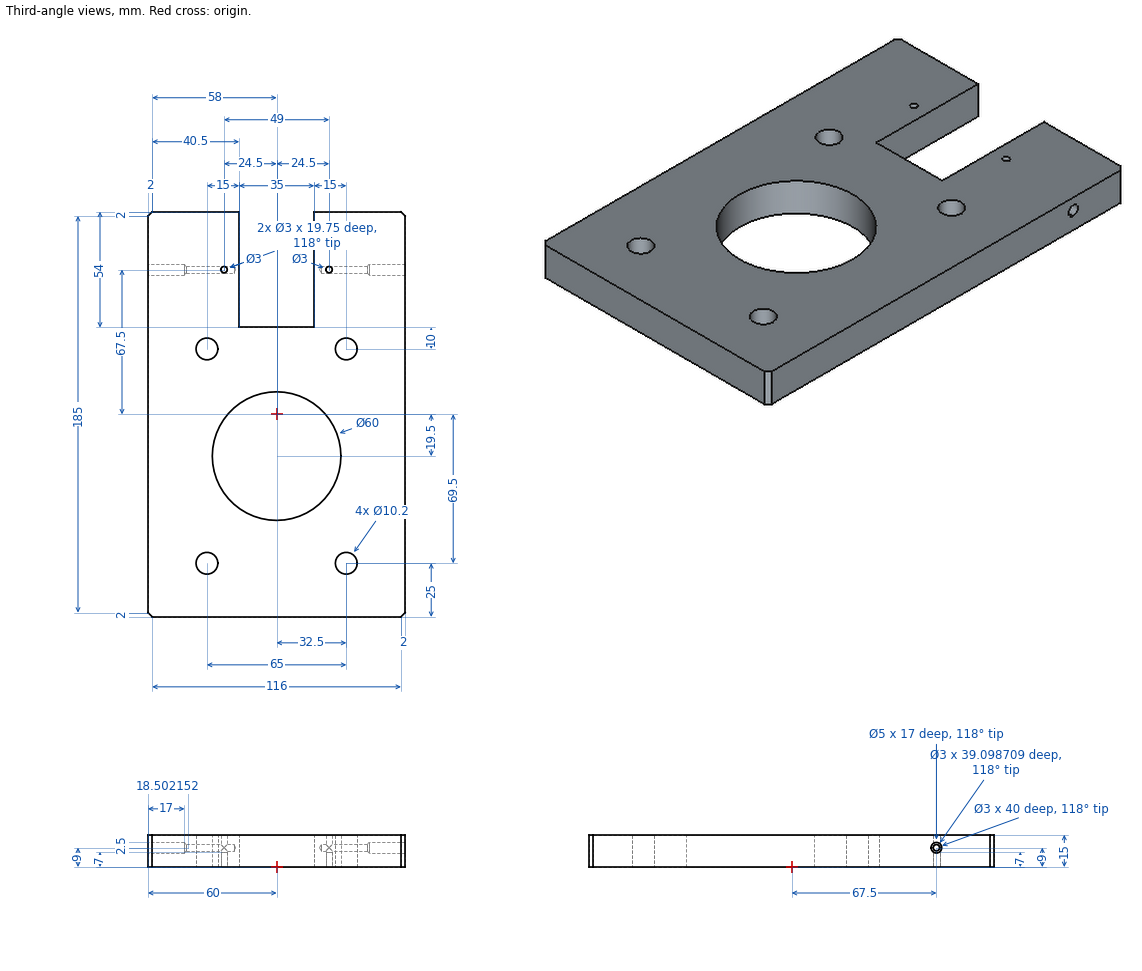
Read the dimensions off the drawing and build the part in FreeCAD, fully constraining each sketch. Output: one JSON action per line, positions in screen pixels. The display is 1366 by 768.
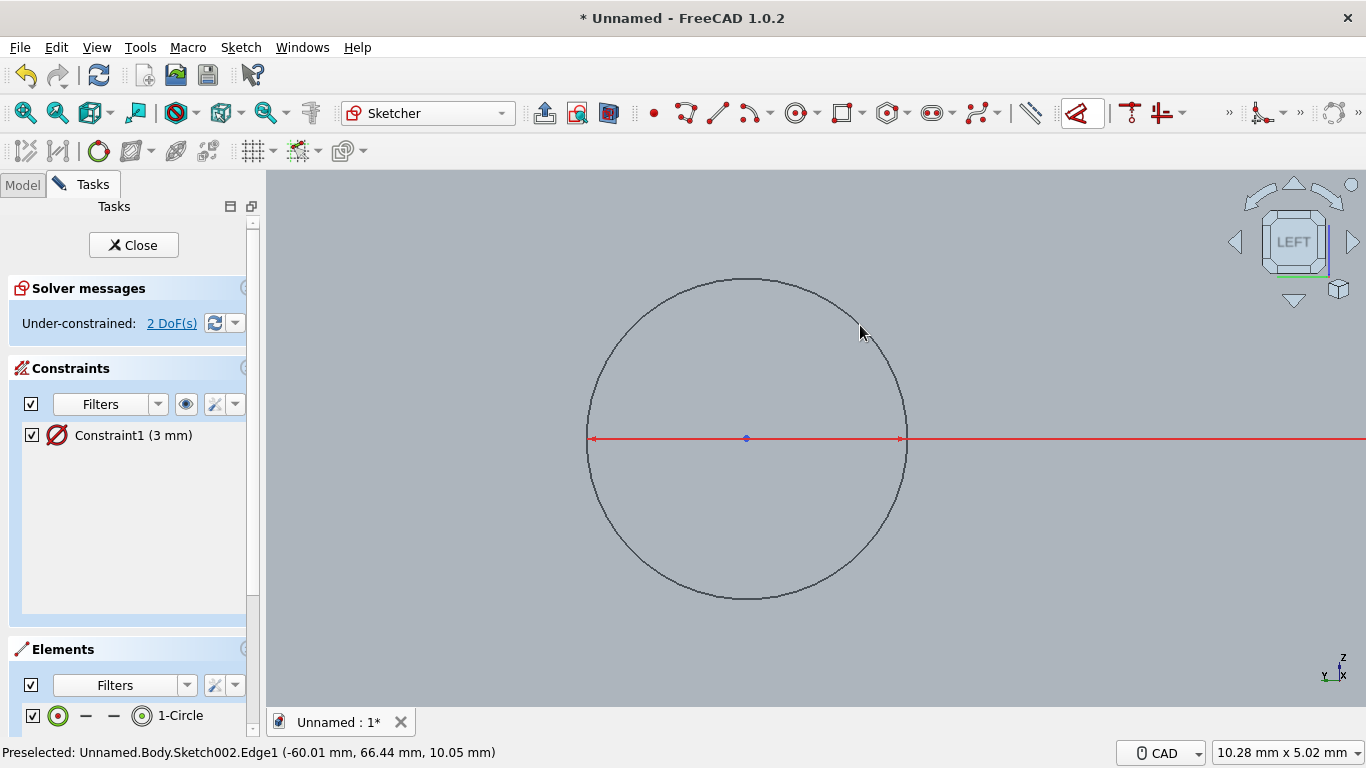
{"action": "left_click", "coordinate": [747, 439]}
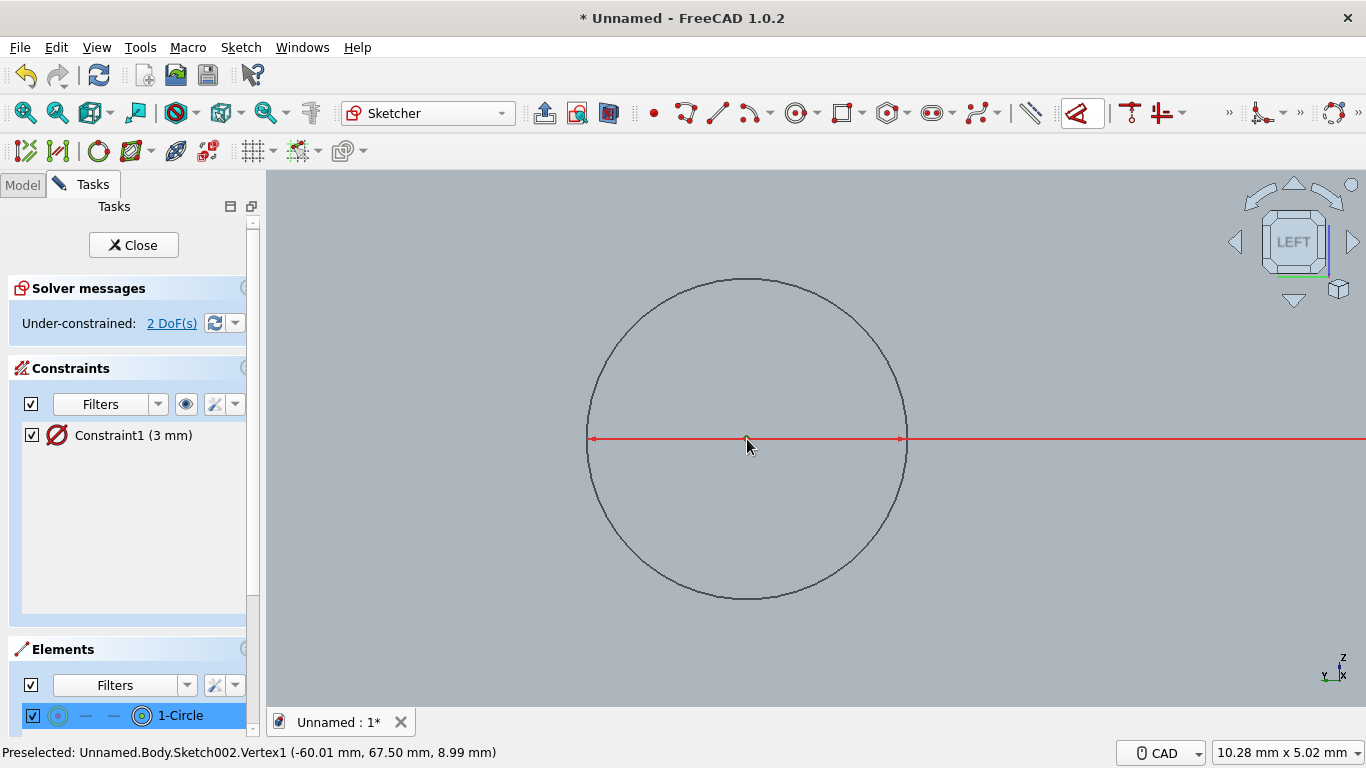
{"action": "left_click", "coordinate": [1098, 114]}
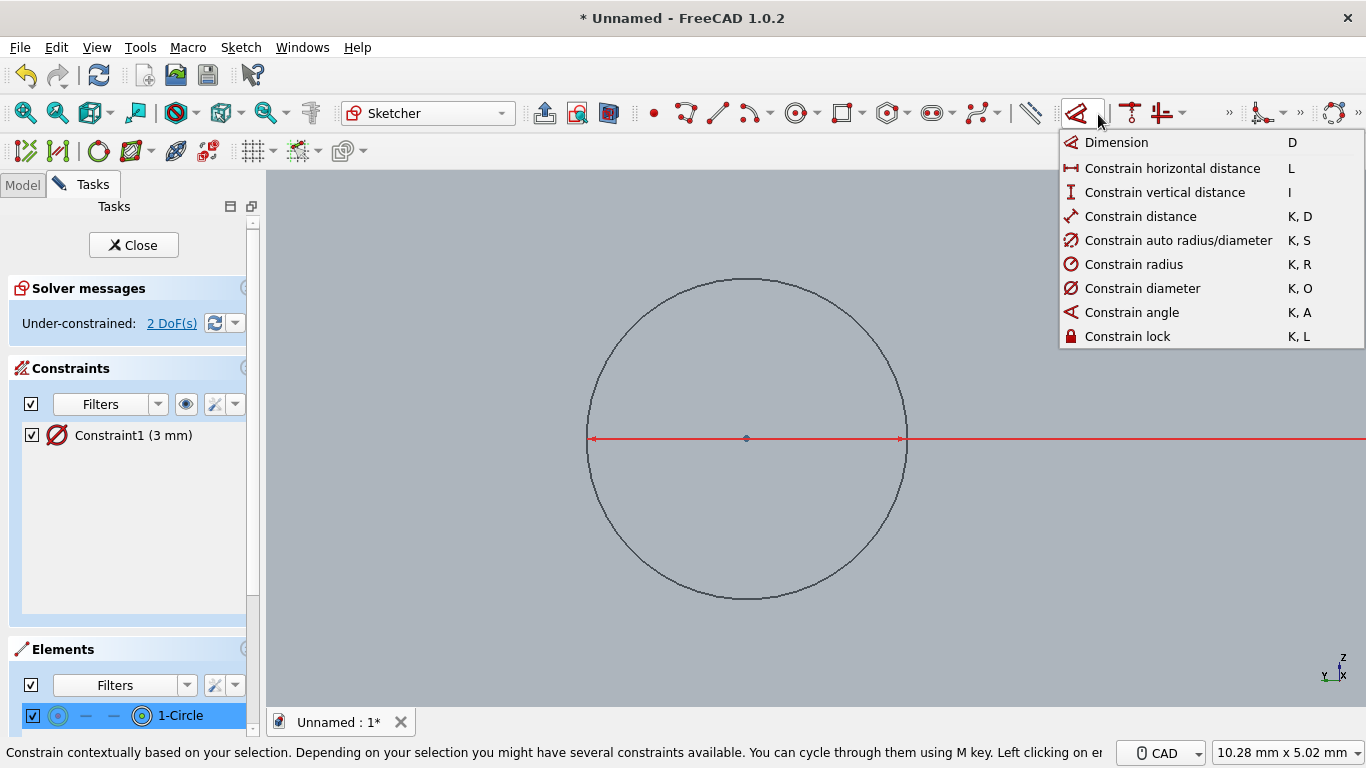
{"action": "left_click", "coordinate": [1212, 192]}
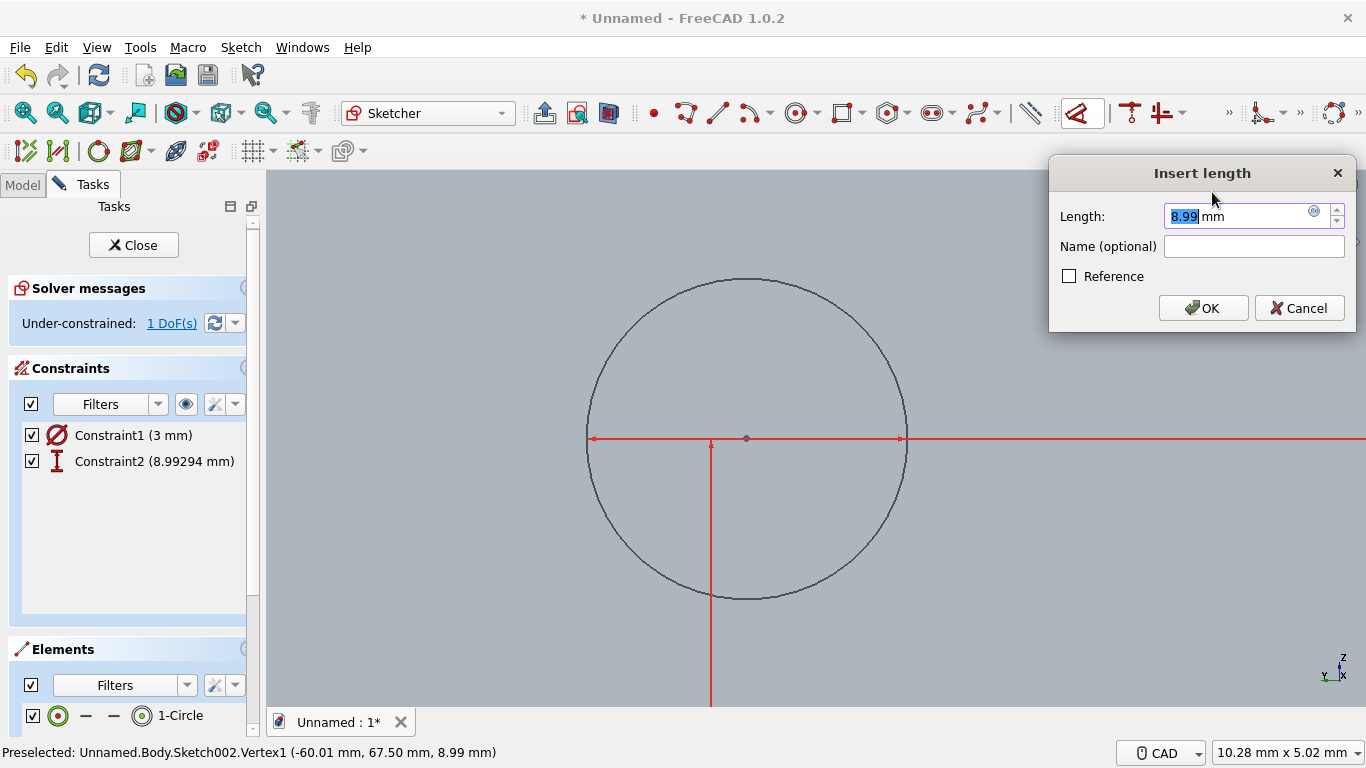
{"action": "type", "text": "9"}
{"action": "key", "text": "Return"}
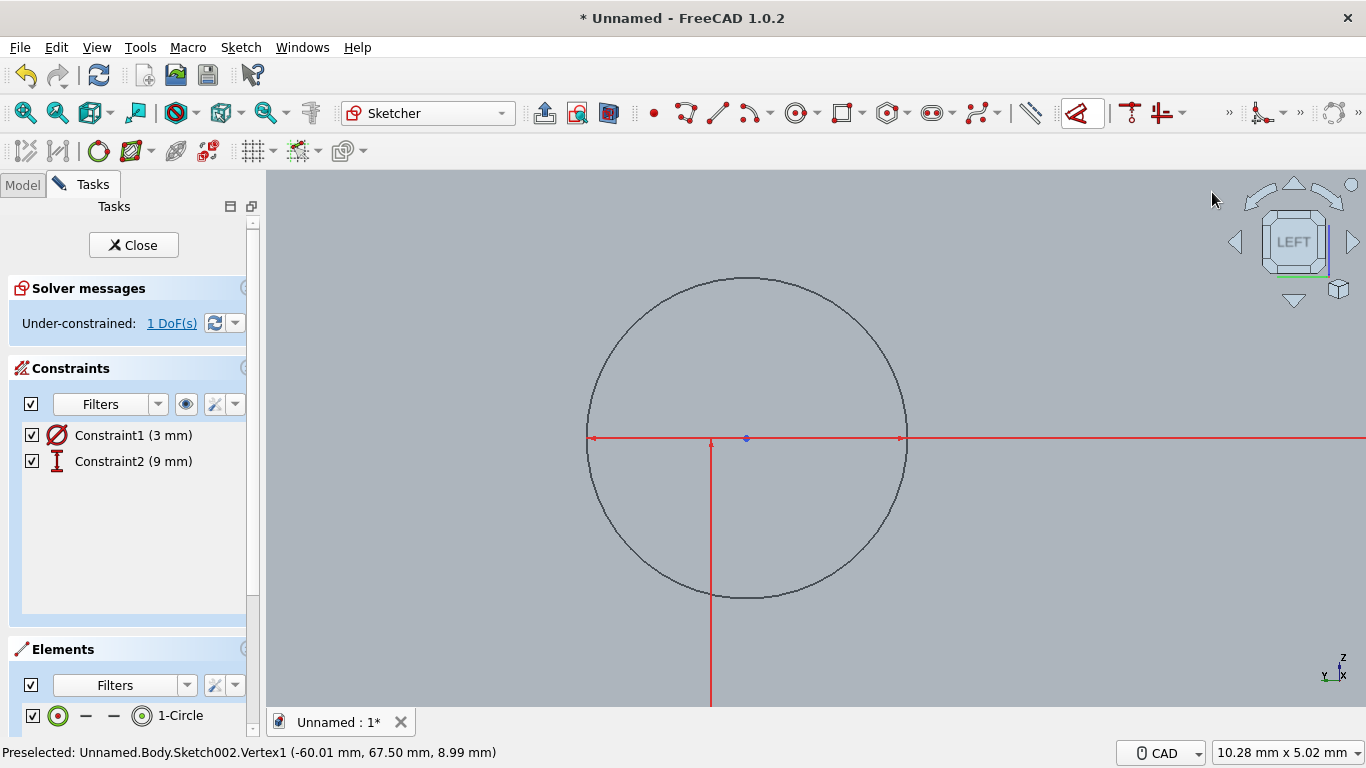
{"action": "left_click", "coordinate": [747, 438]}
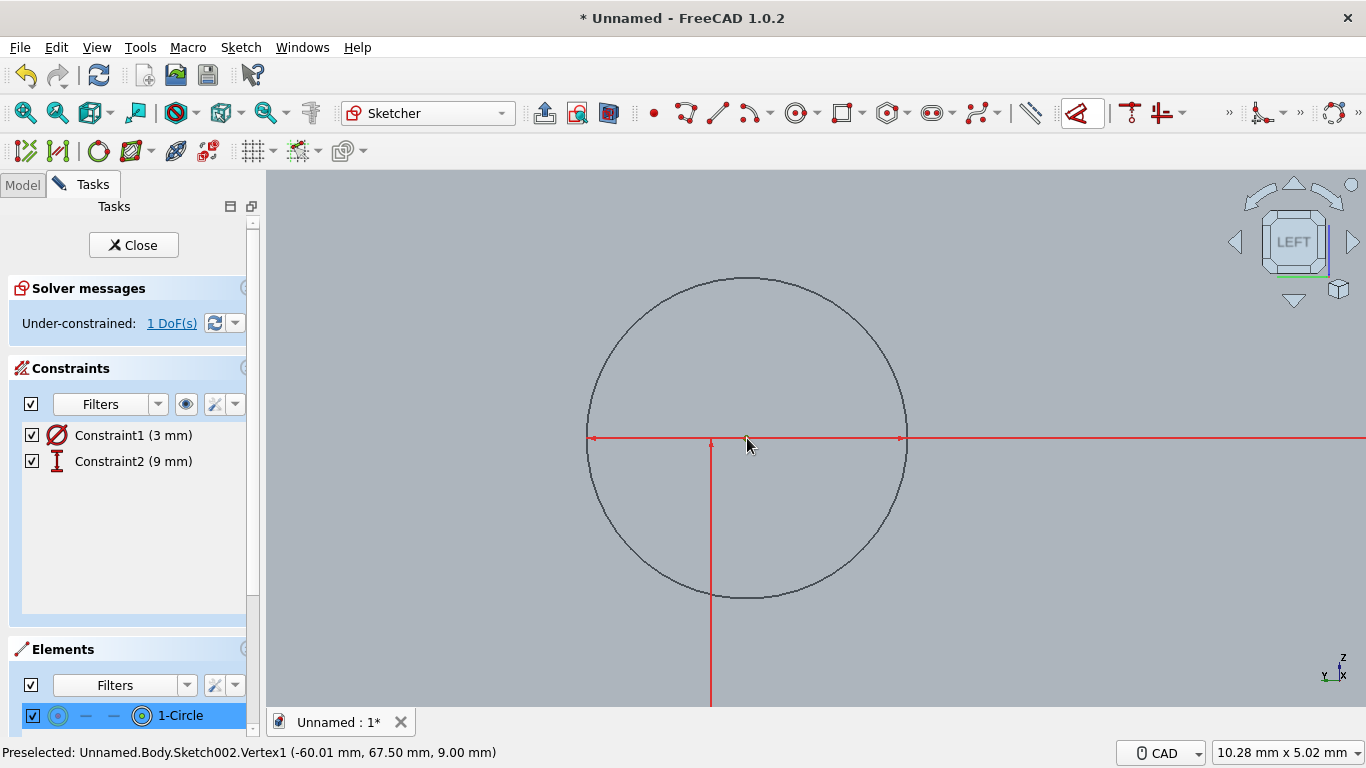
{"action": "key", "text": "l"}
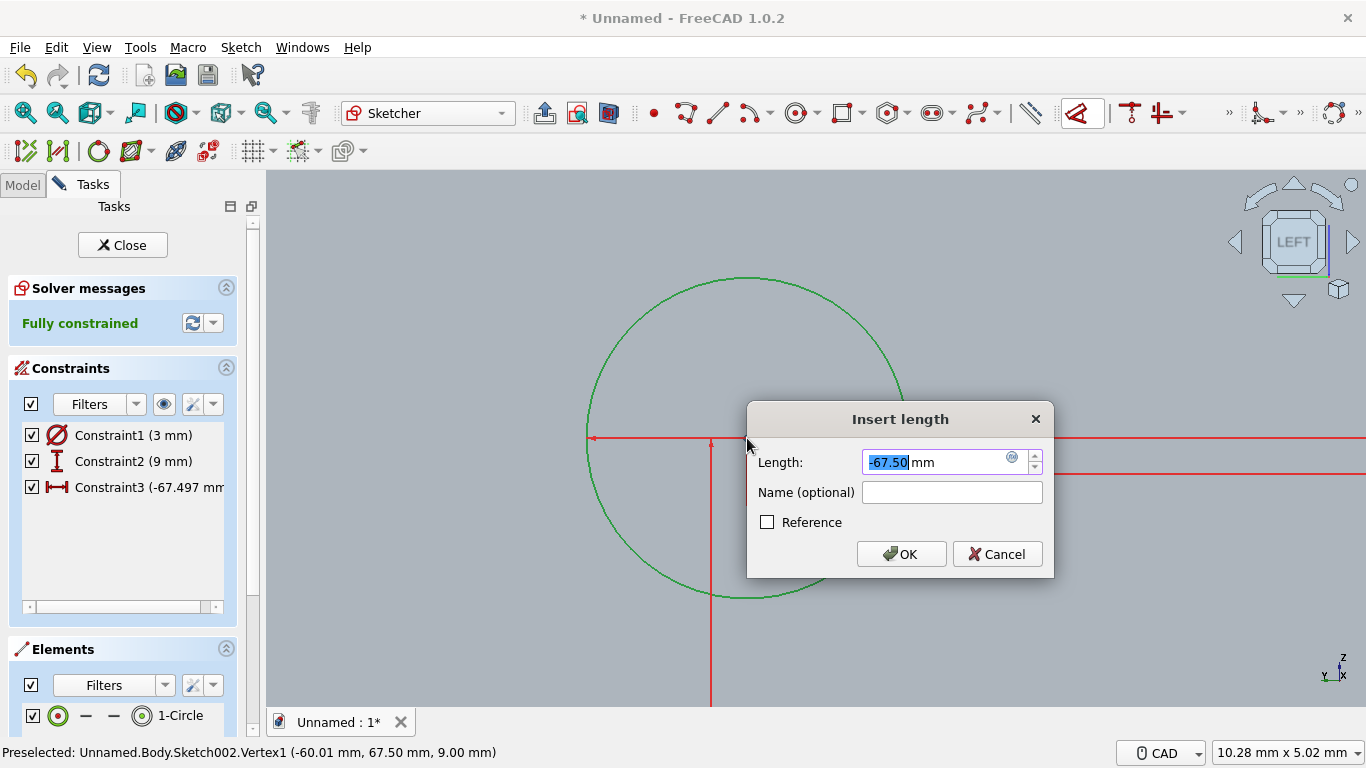
{"action": "type", "text": "-67.5"}
{"action": "key", "text": "Return"}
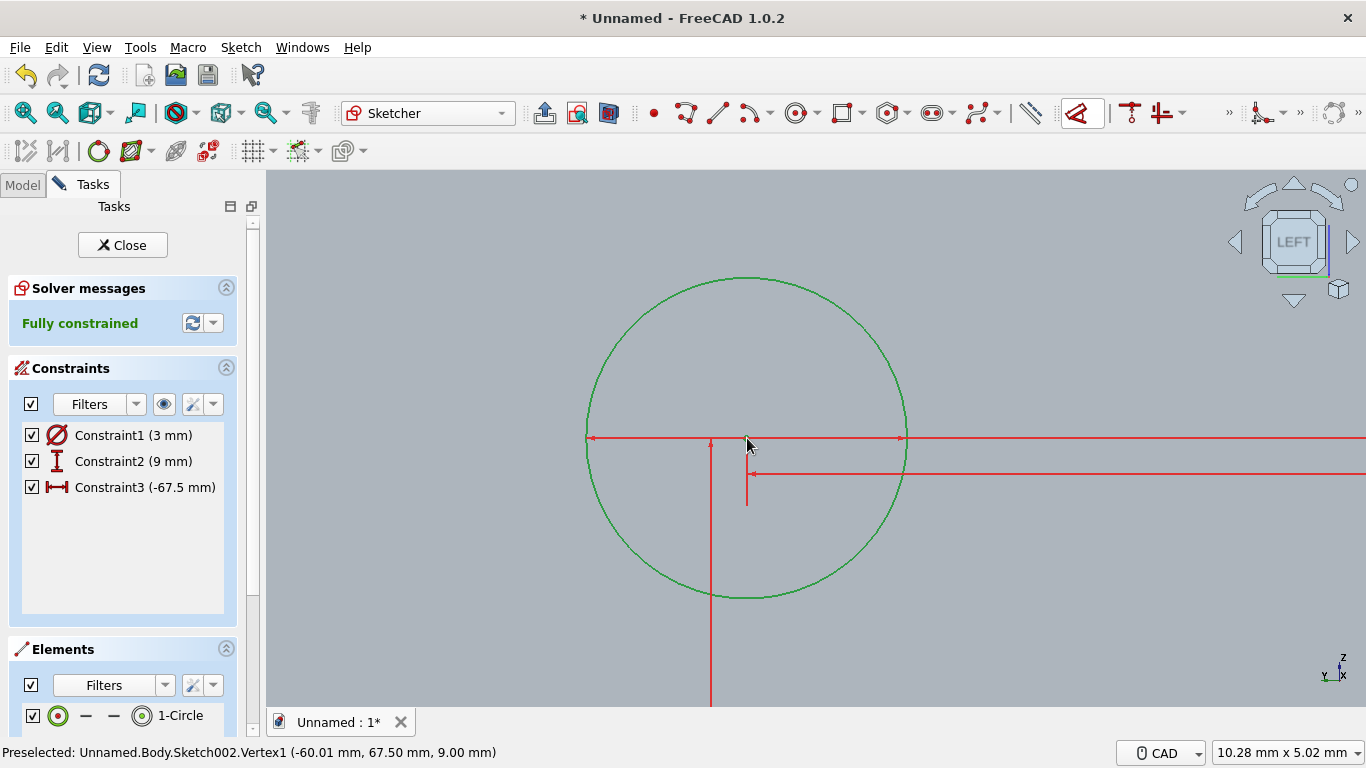
{"action": "left_click", "coordinate": [123, 245]}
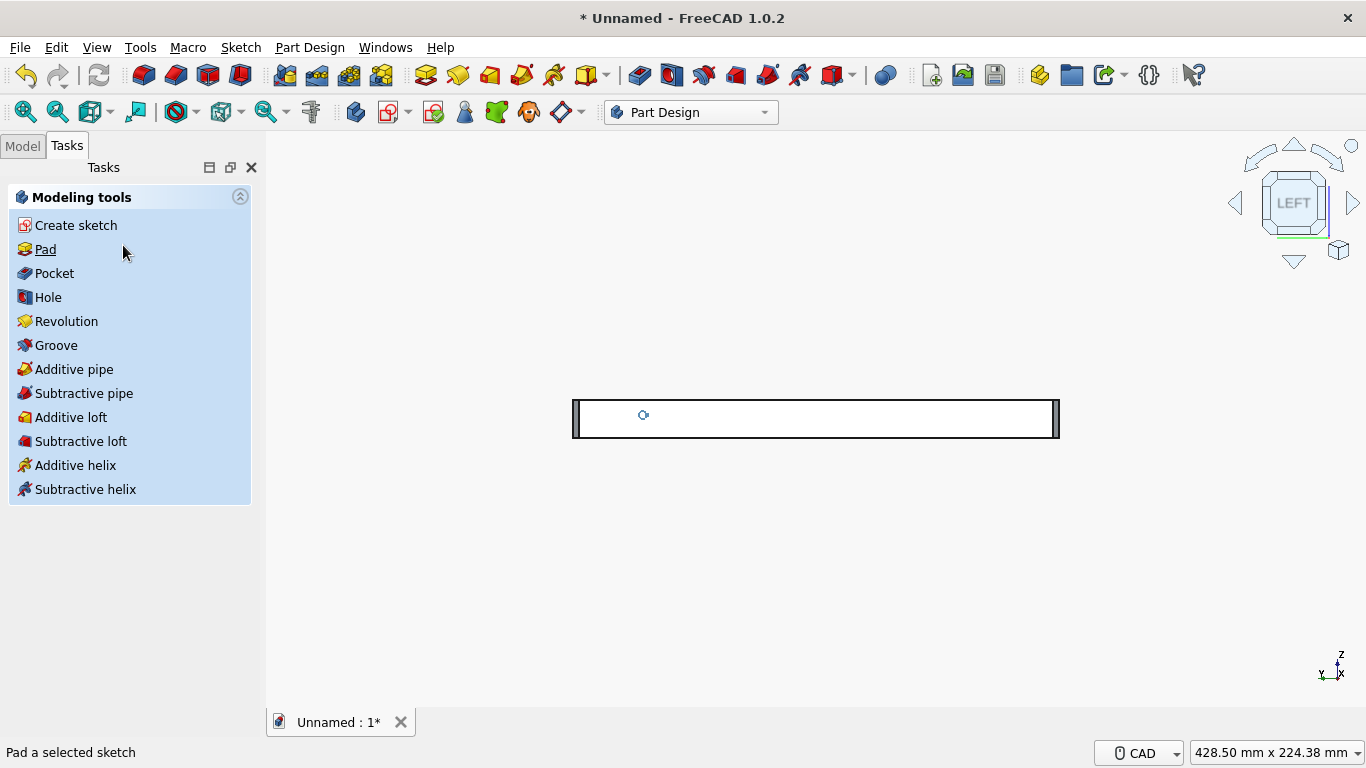
{"action": "left_click", "coordinate": [672, 76]}